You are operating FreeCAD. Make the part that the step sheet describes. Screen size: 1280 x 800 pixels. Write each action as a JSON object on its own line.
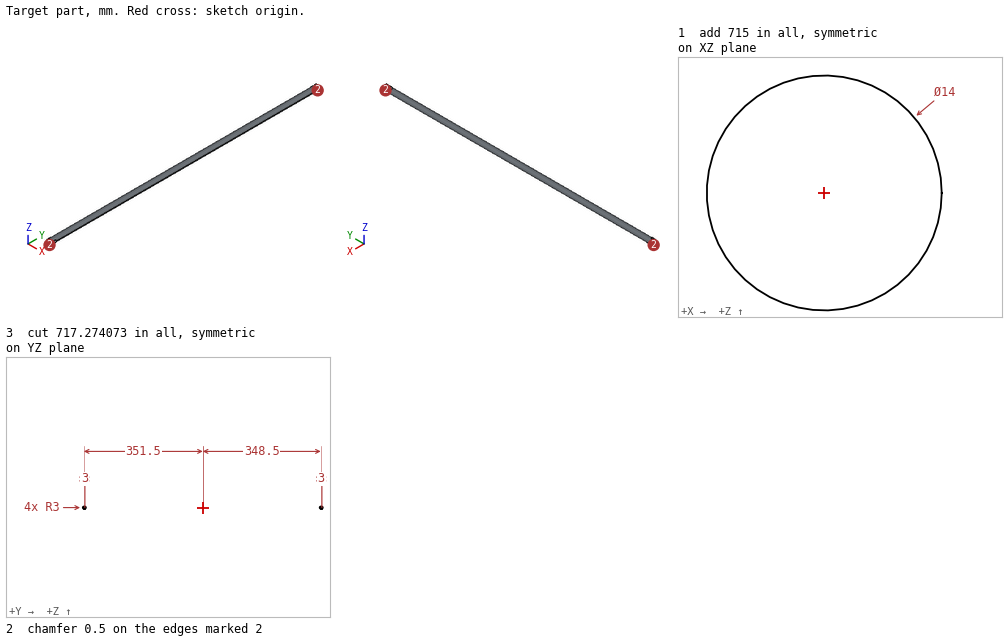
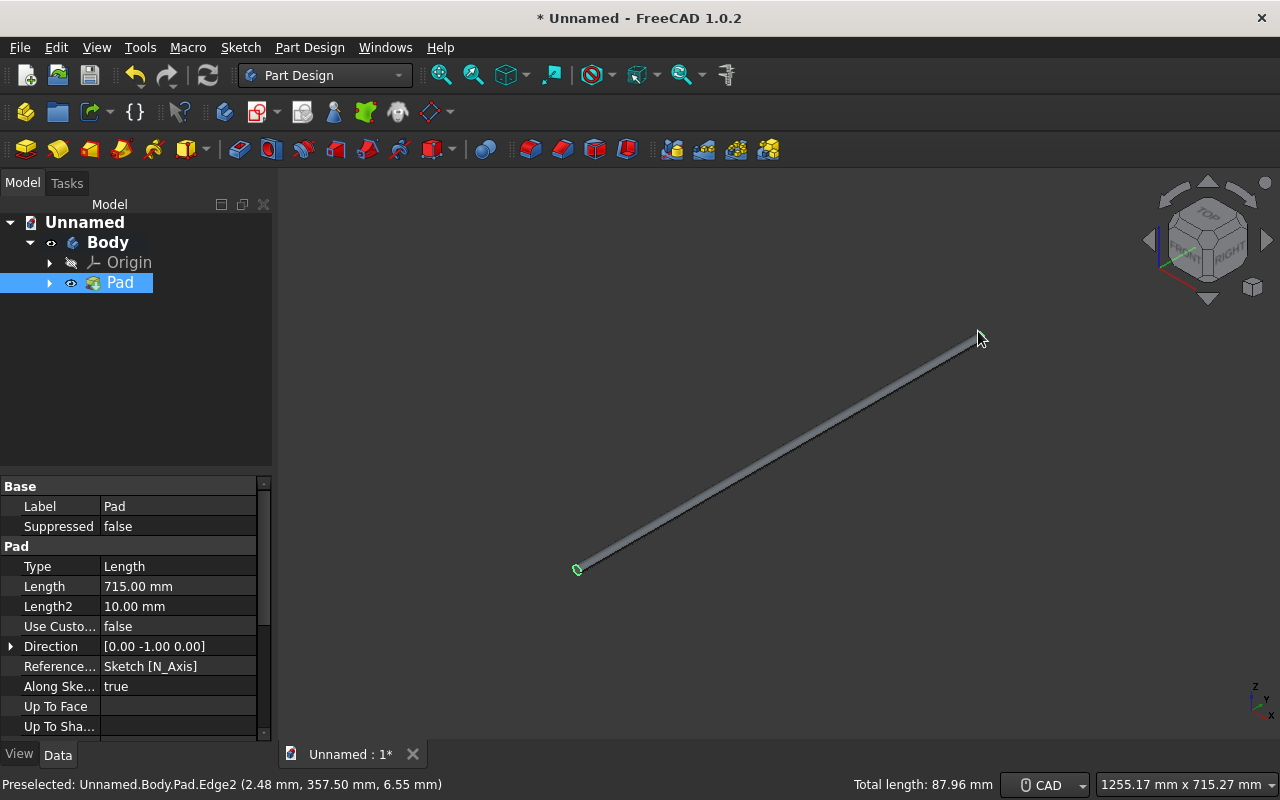
{"action": "left_click", "coordinate": [564, 150]}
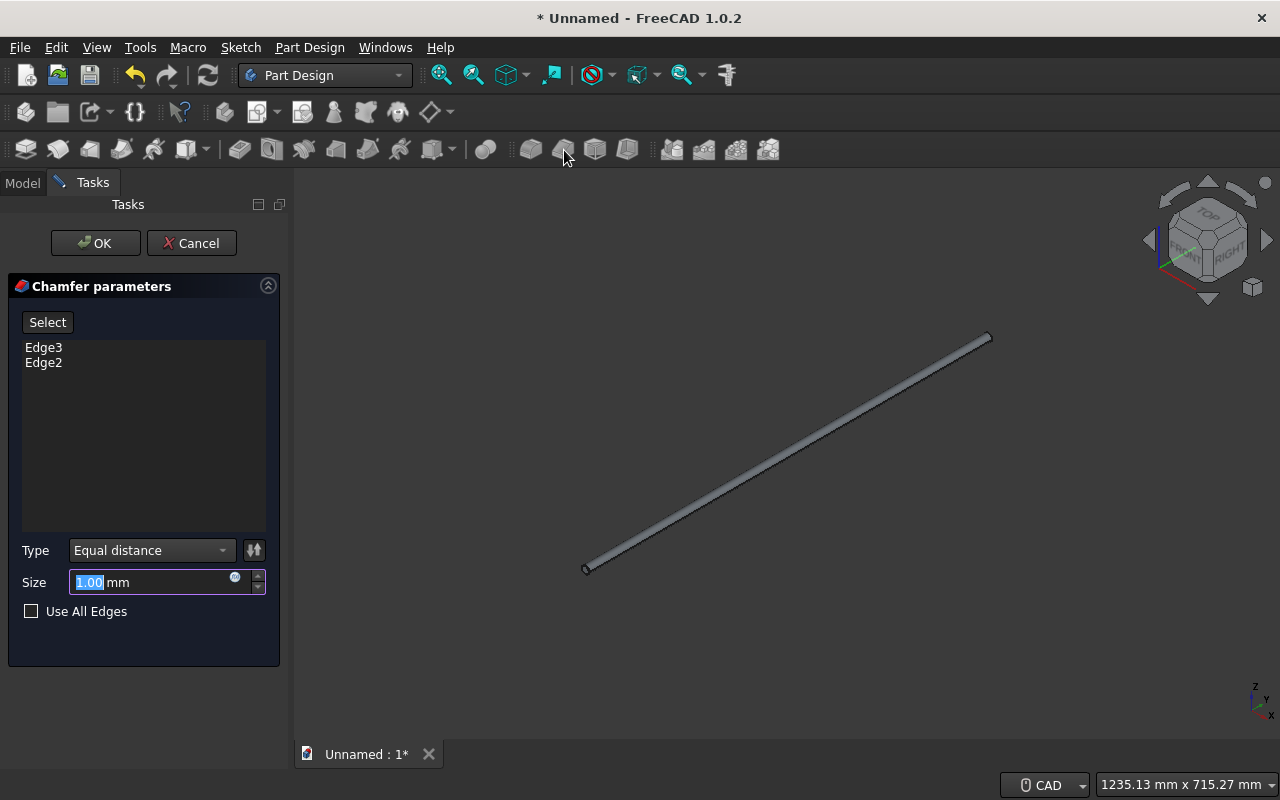
{"action": "type", "text": "0.5"}
{"action": "key", "text": "Tab"}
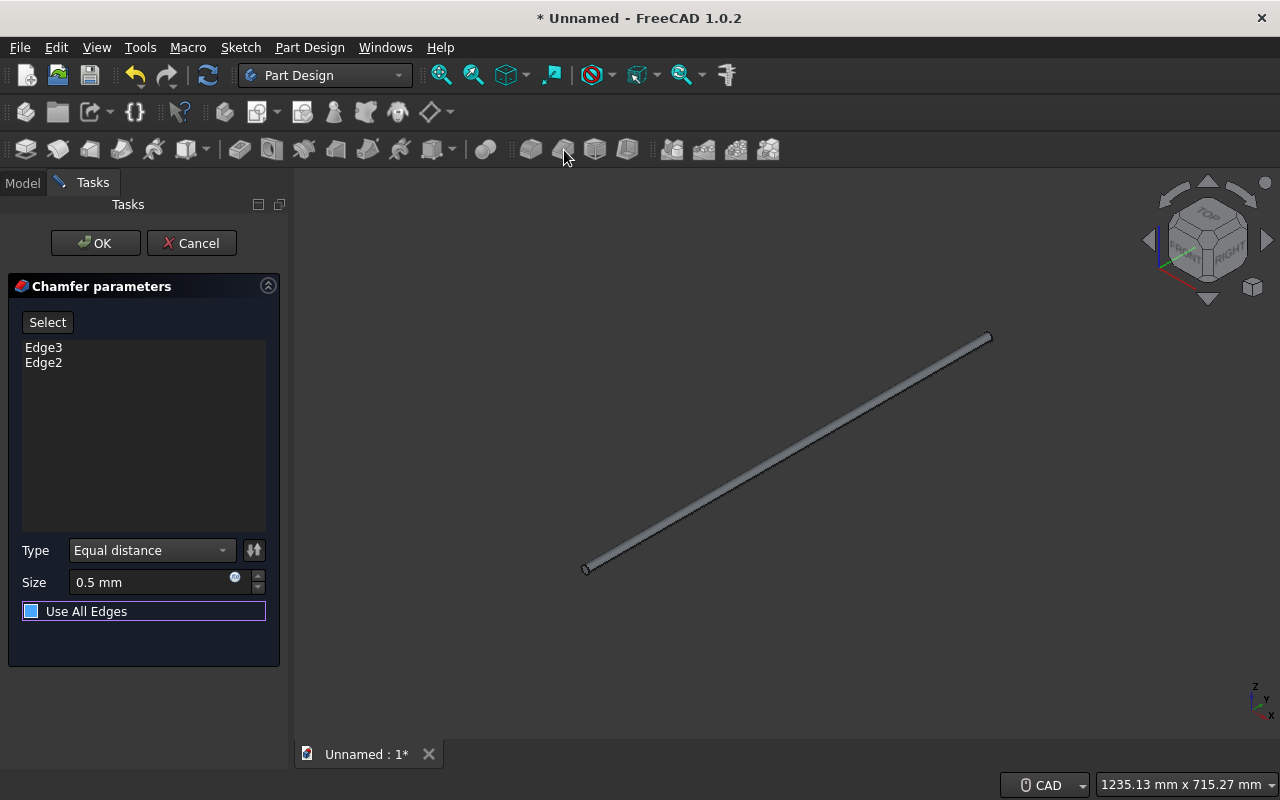
{"action": "left_click", "coordinate": [96, 243]}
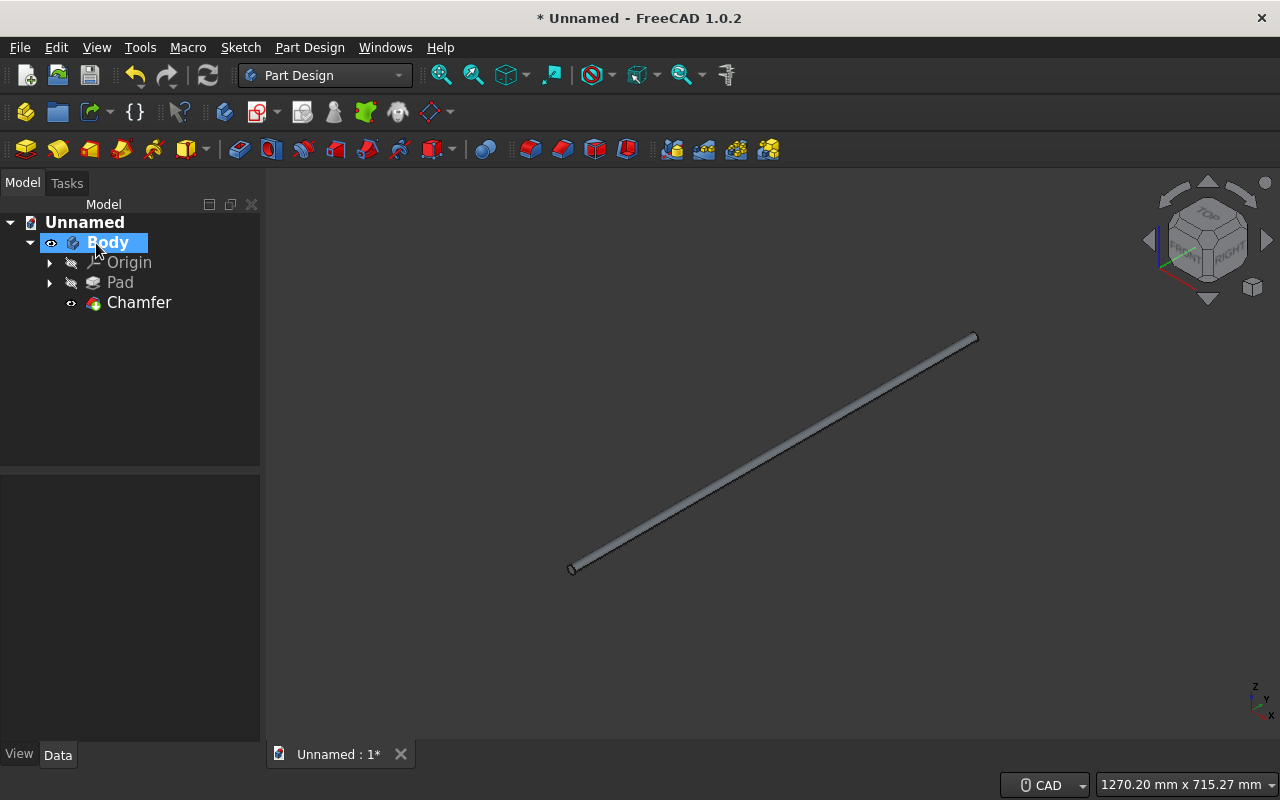
{"action": "left_click", "coordinate": [442, 76]}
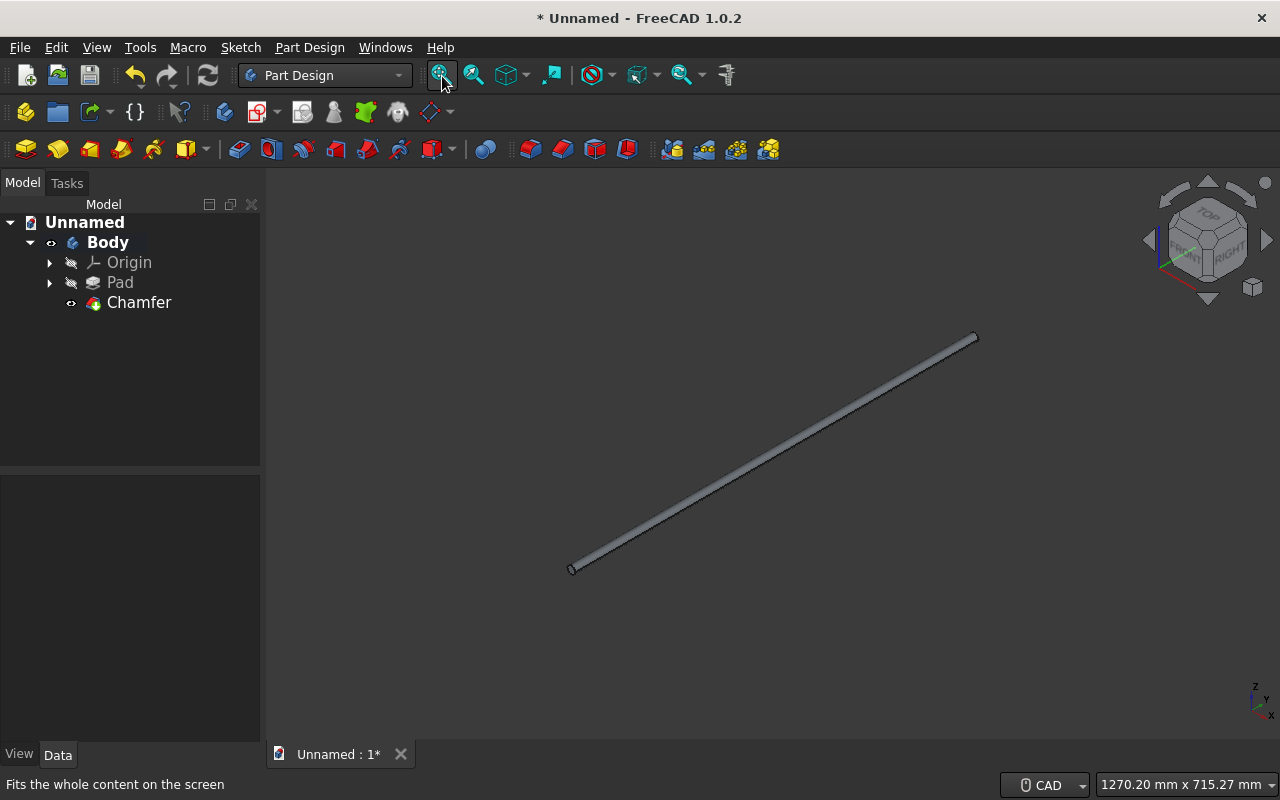
{"action": "left_click", "coordinate": [258, 112]}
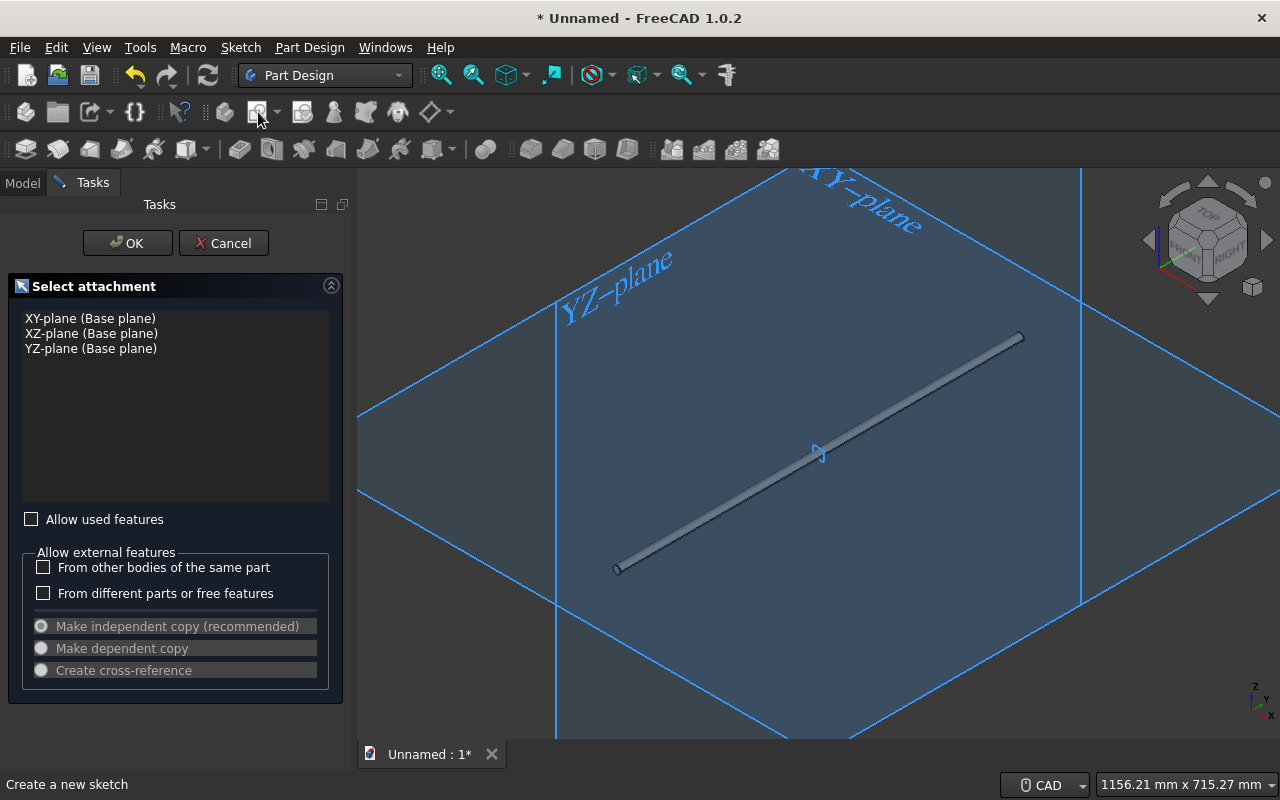
{"action": "left_click", "coordinate": [82, 348]}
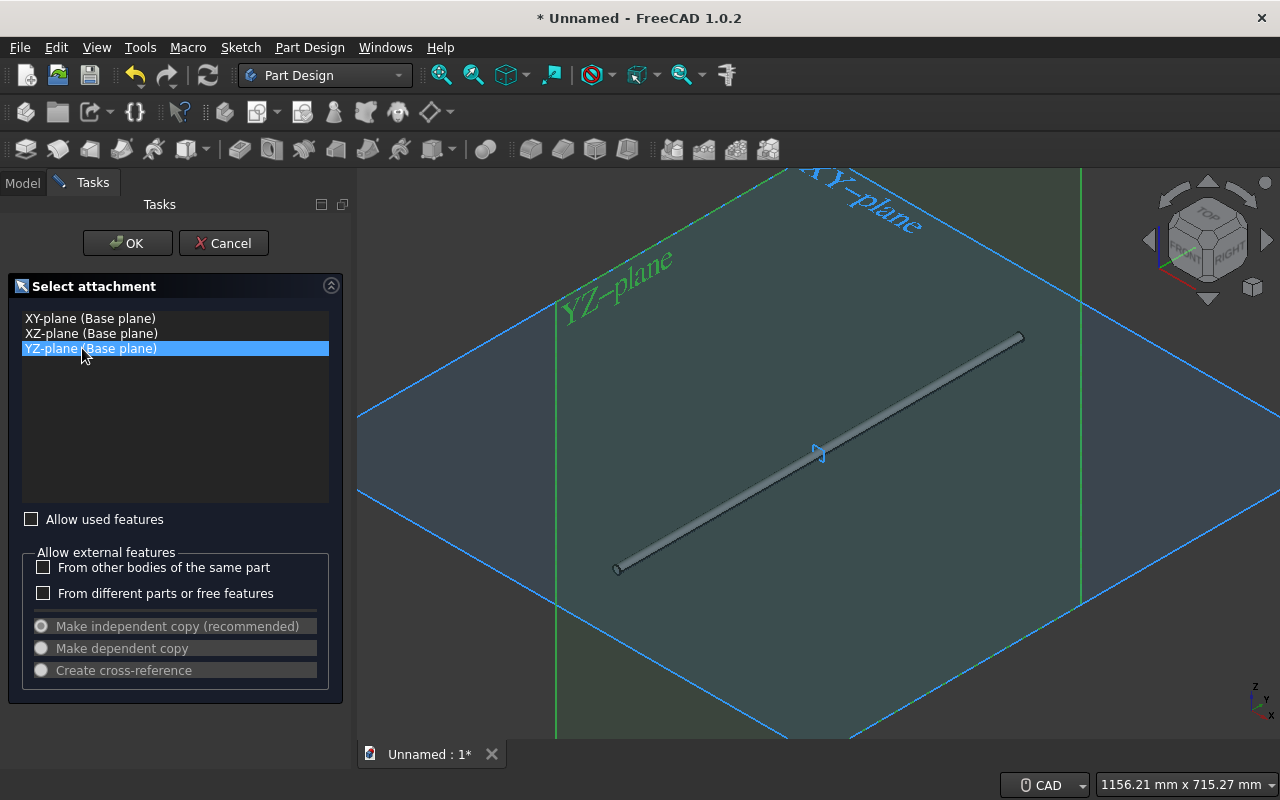
{"action": "left_click", "coordinate": [128, 243]}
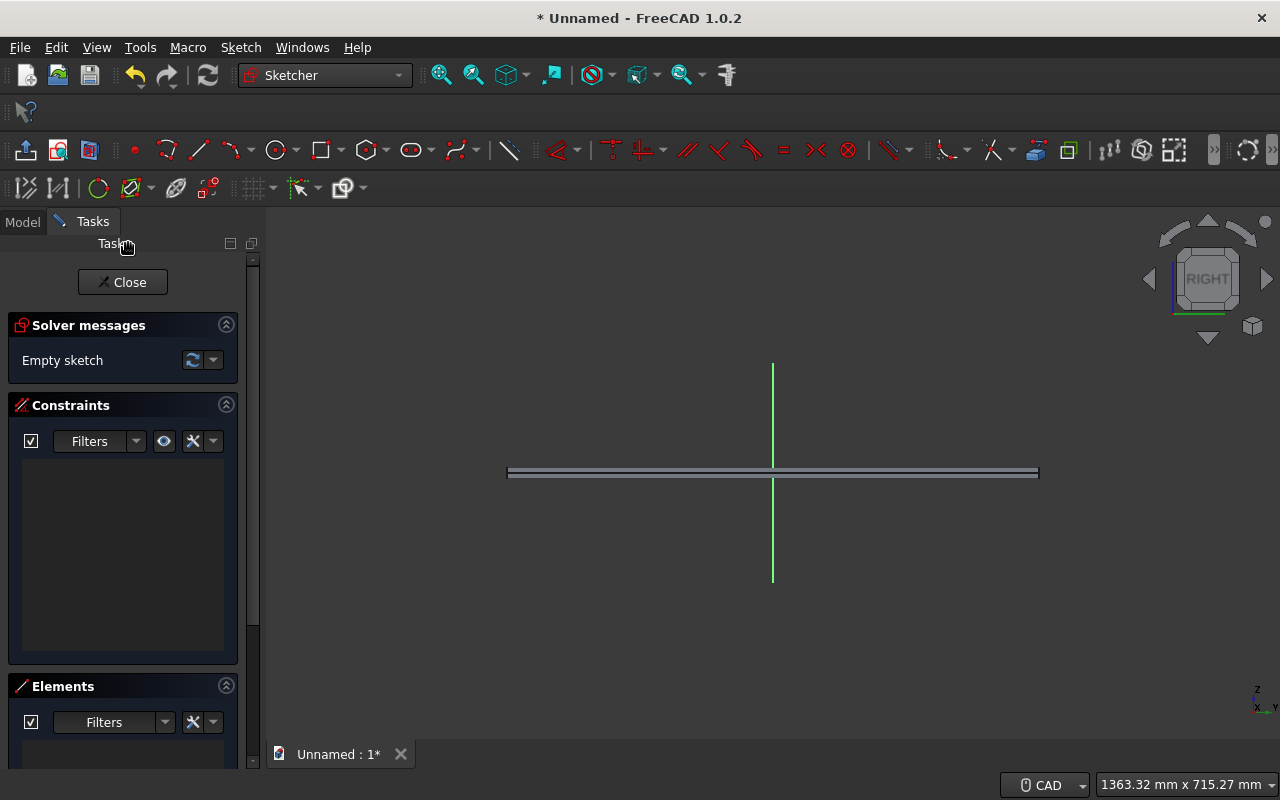
{"action": "left_click", "coordinate": [90, 150]}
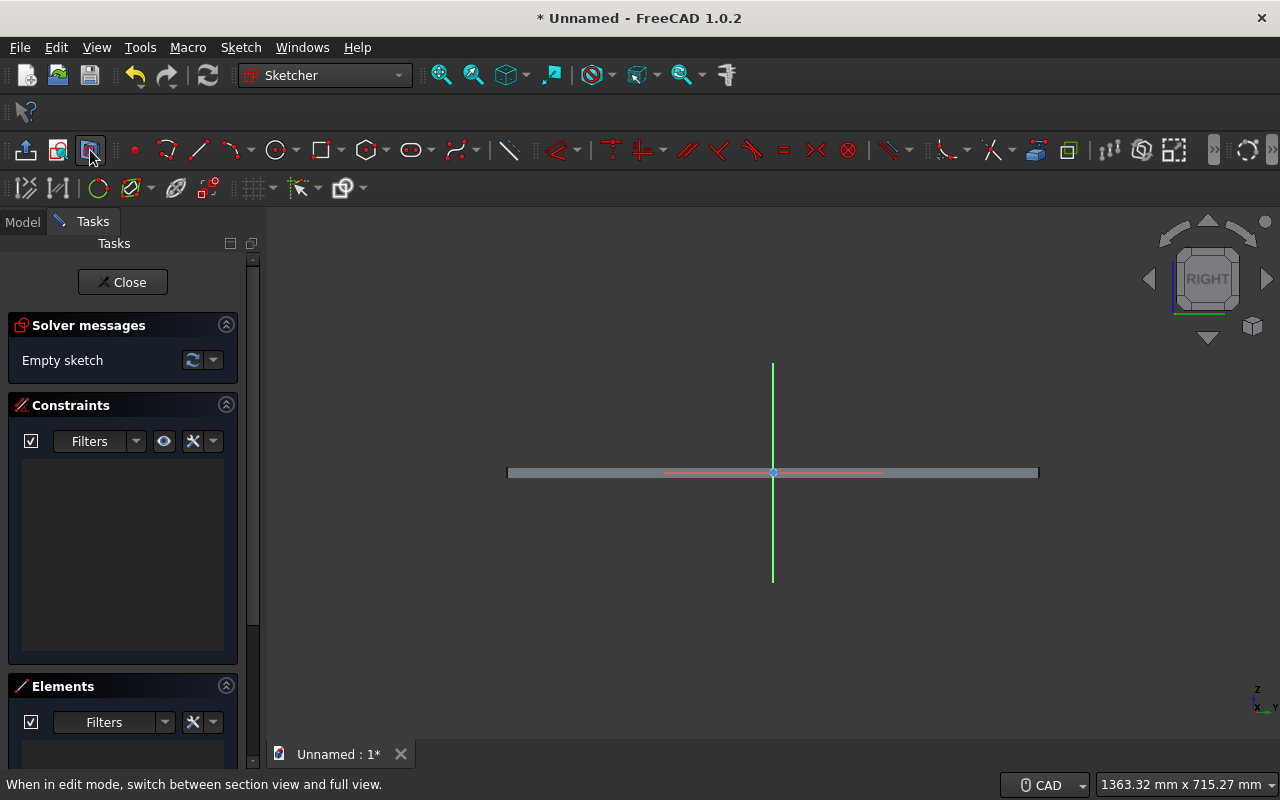
{"action": "left_click", "coordinate": [412, 150]}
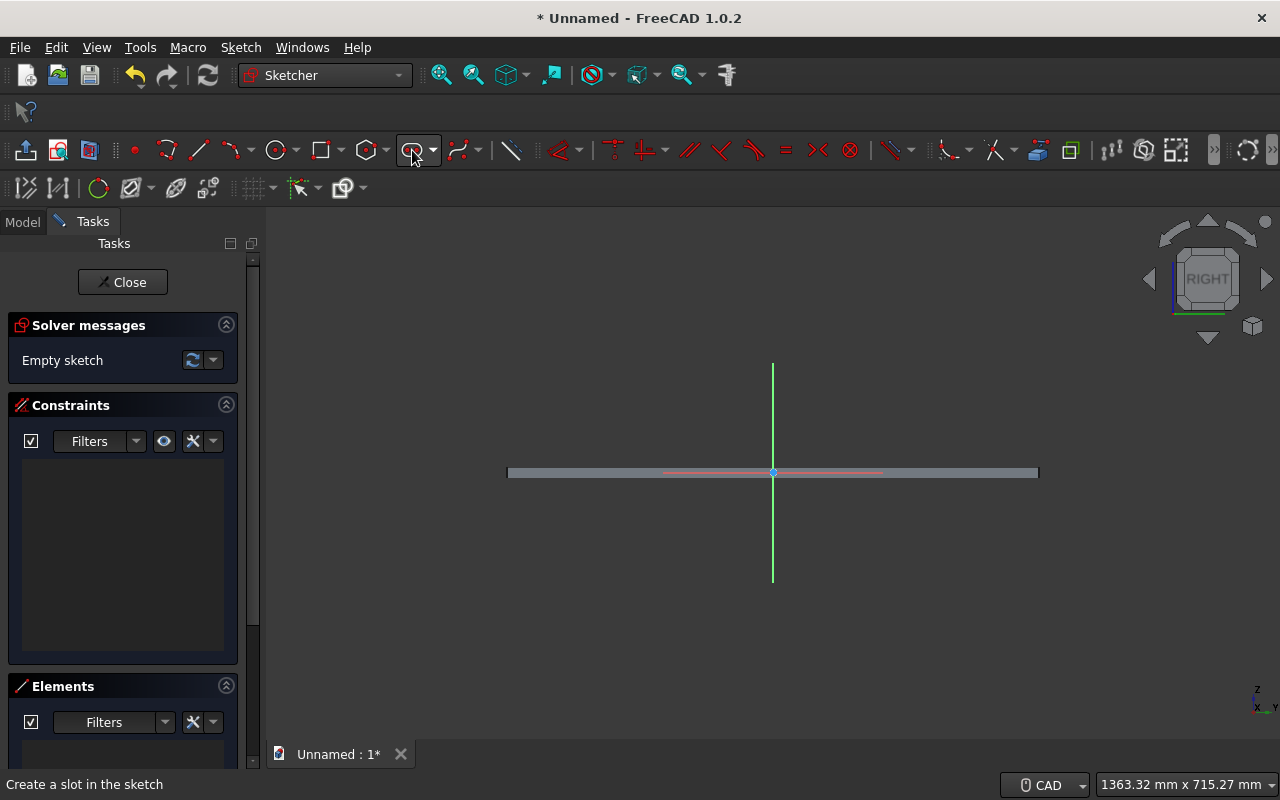
{"action": "scroll", "coordinate": [512, 473], "scroll_direction": "up", "scroll_amount": 12}